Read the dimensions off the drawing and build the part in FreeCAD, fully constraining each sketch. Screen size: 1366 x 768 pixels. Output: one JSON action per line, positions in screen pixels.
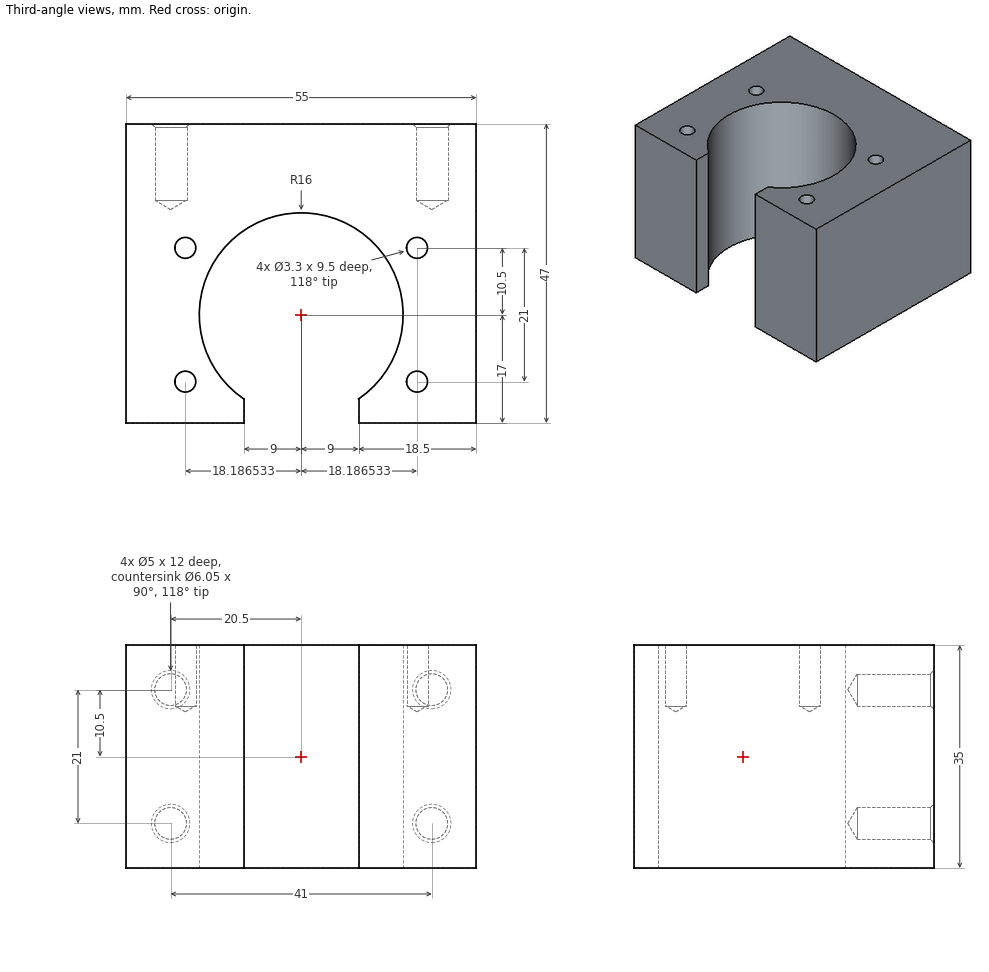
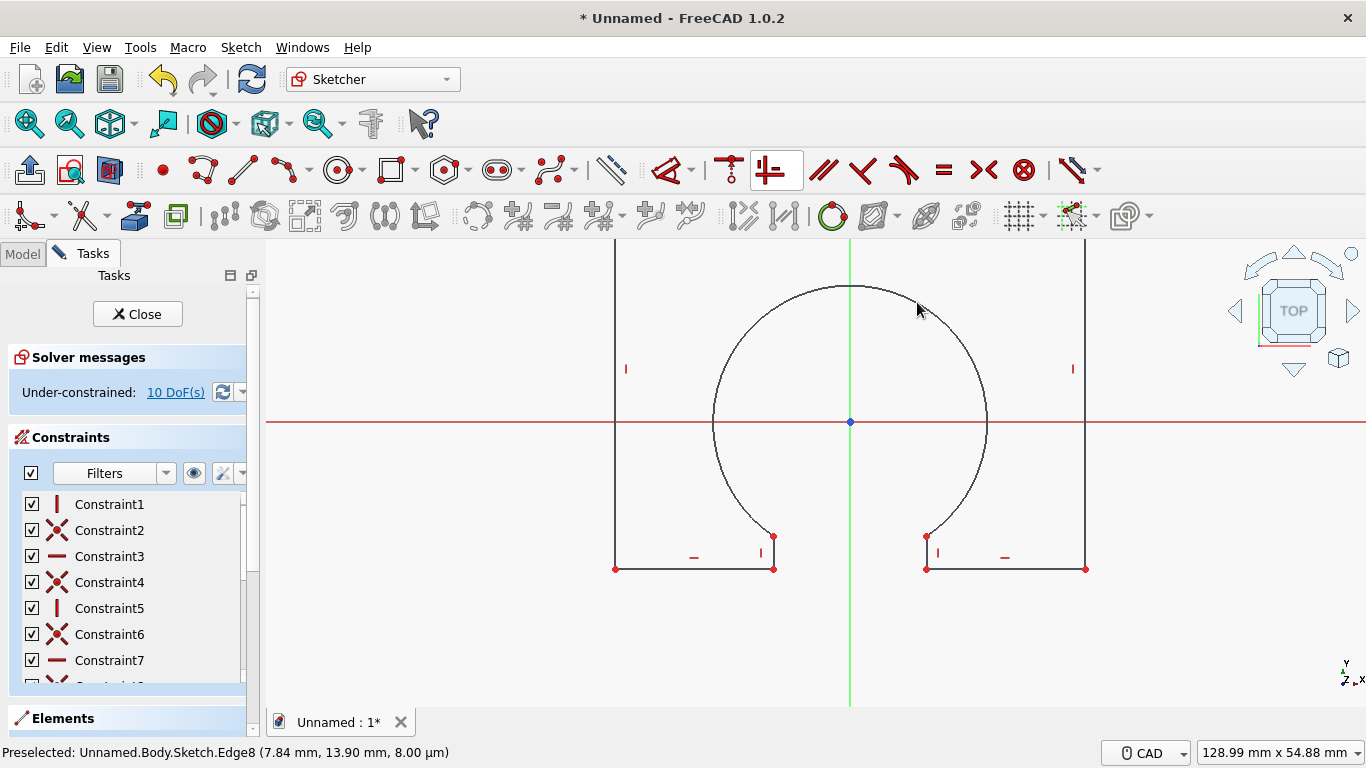
{"action": "left_click_drag", "start_coordinate": [840, 412], "coordinate": [860, 433]}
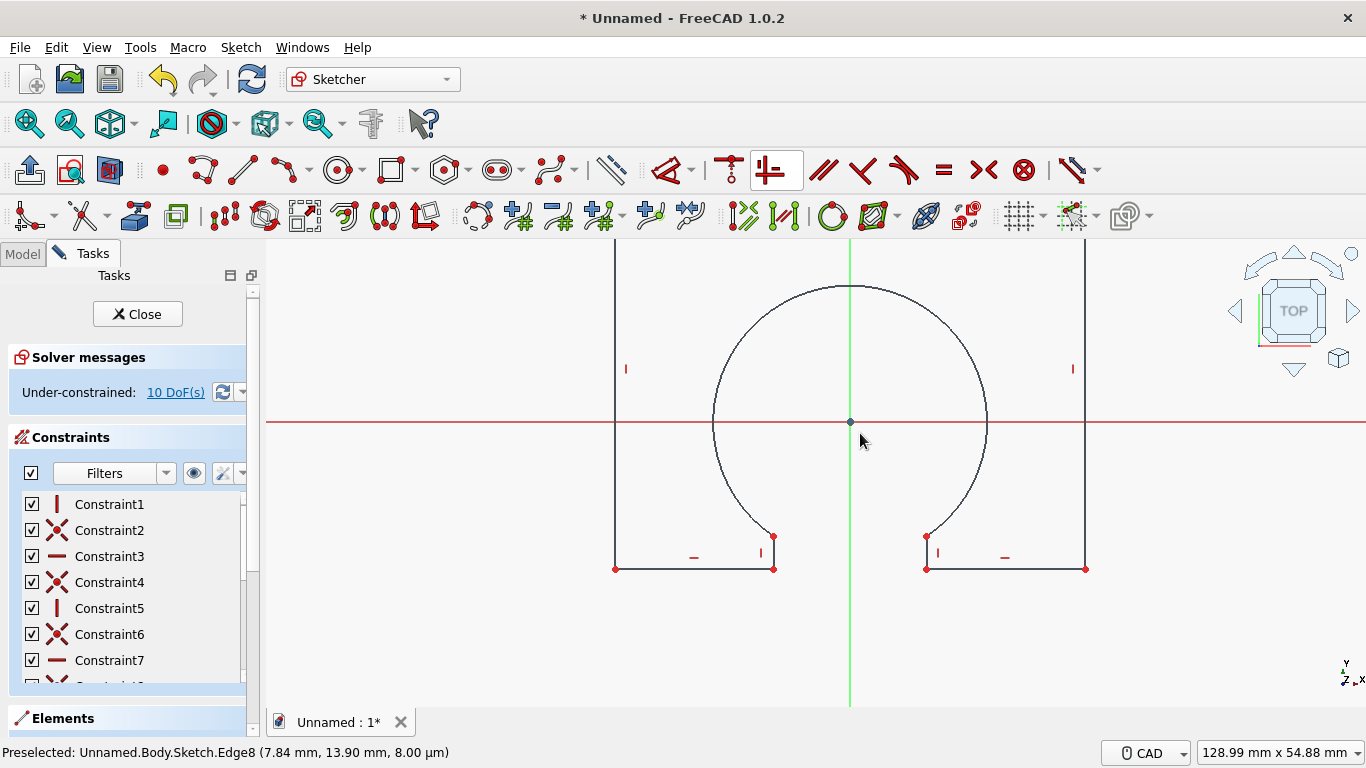
{"action": "left_click", "coordinate": [730, 170]}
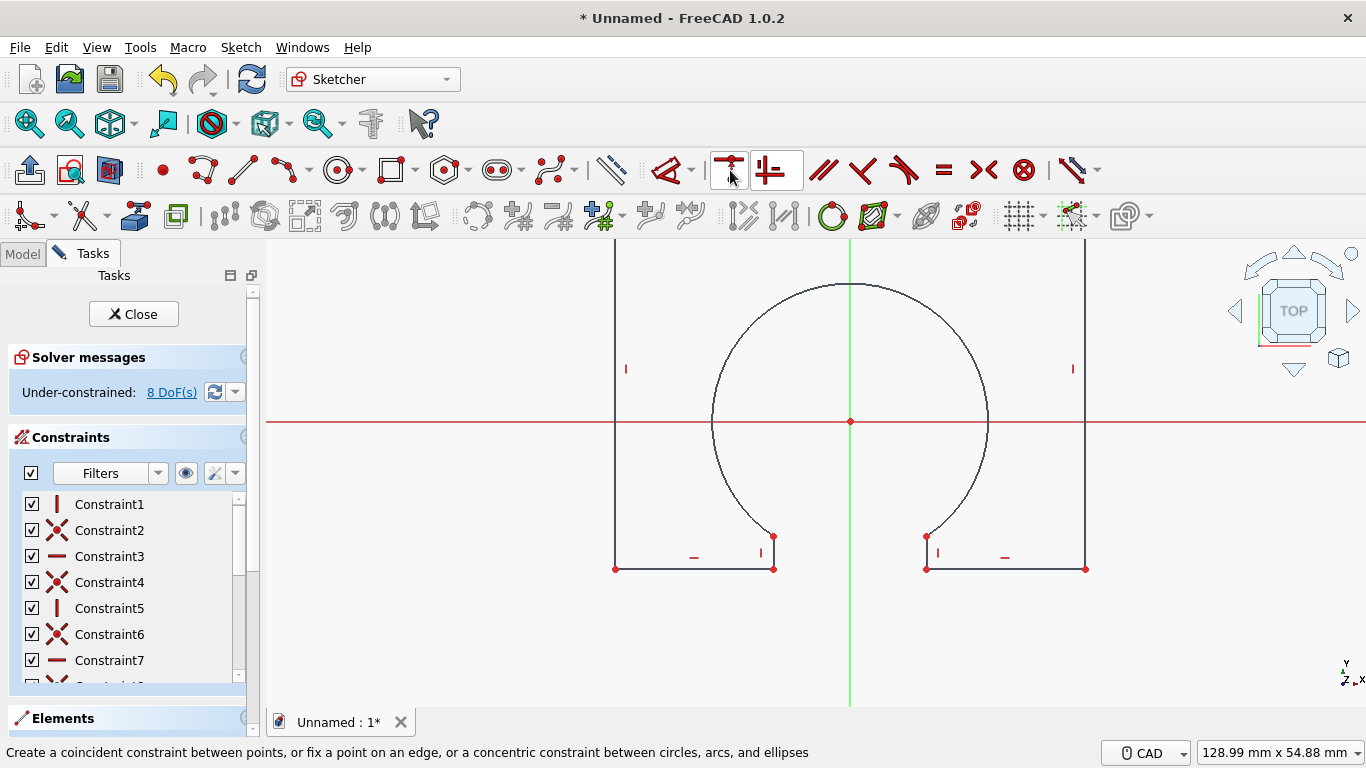
{"action": "left_click", "coordinate": [666, 170]}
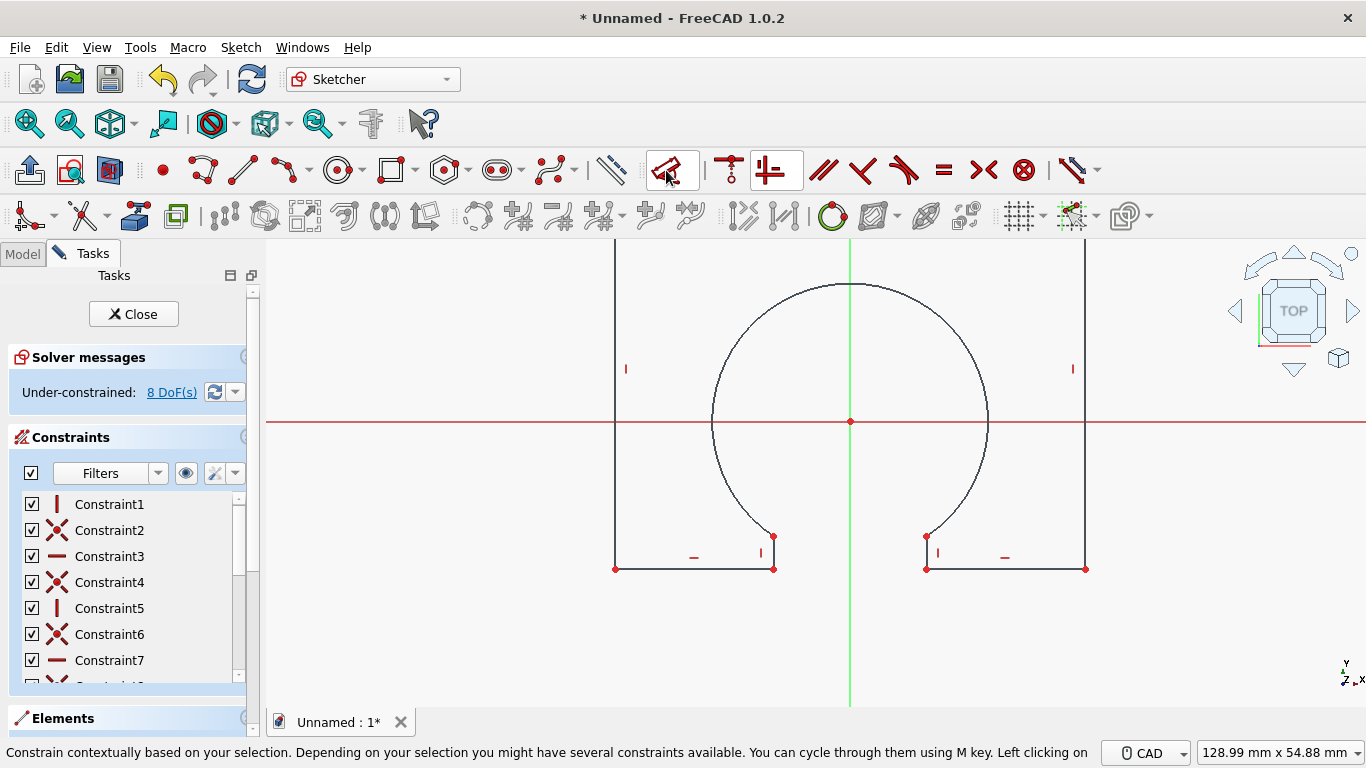
{"action": "left_click", "coordinate": [968, 349]}
{"action": "left_click", "coordinate": [995, 332]}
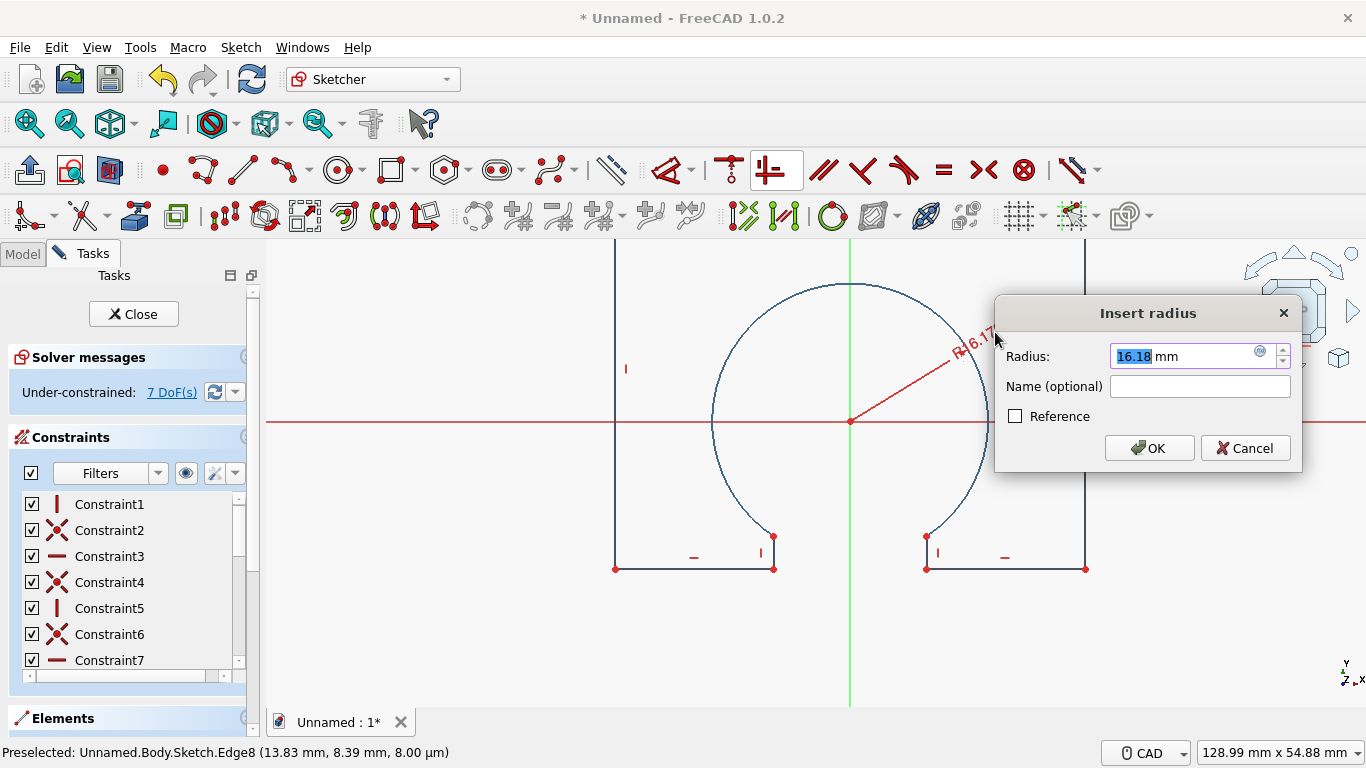
{"action": "type", "text": "16"}
{"action": "key", "text": "Return"}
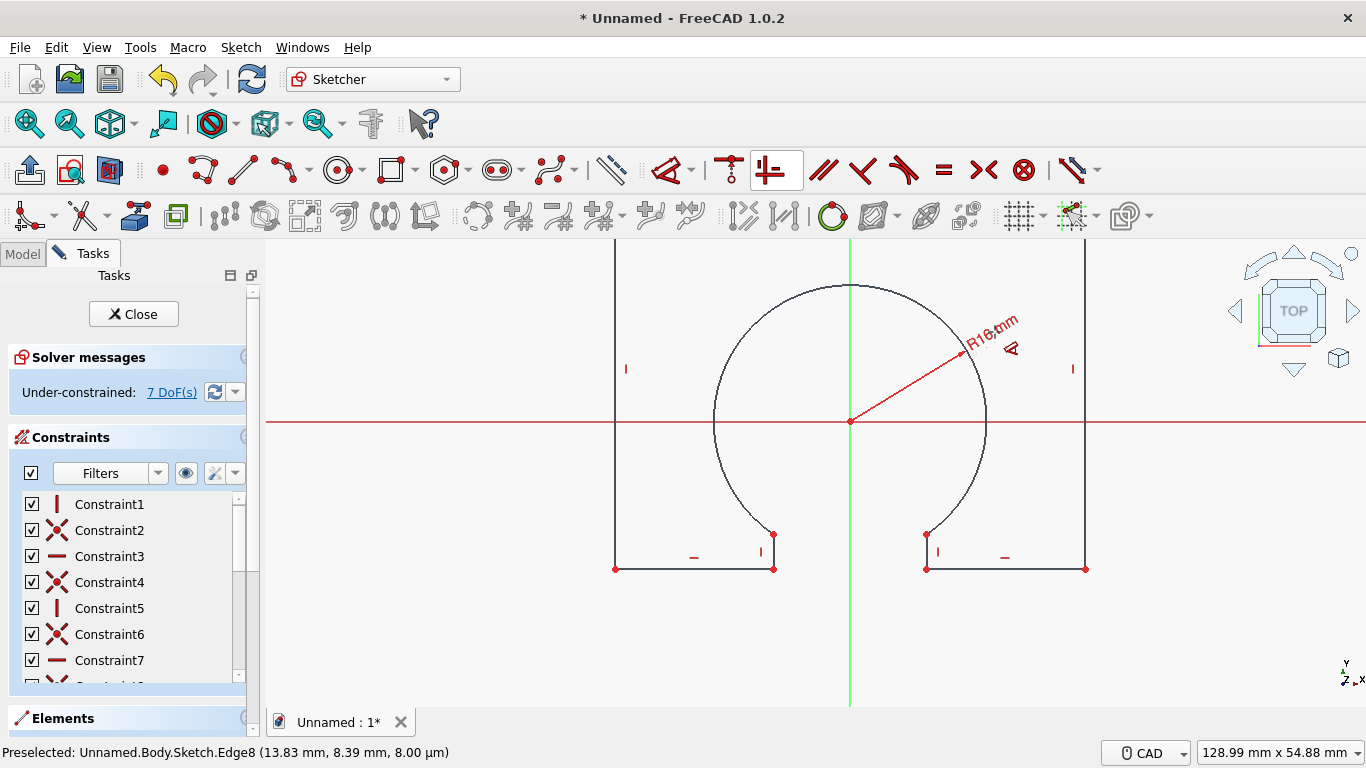
{"action": "left_click", "coordinate": [1085, 449]}
{"action": "left_click", "coordinate": [1119, 349]}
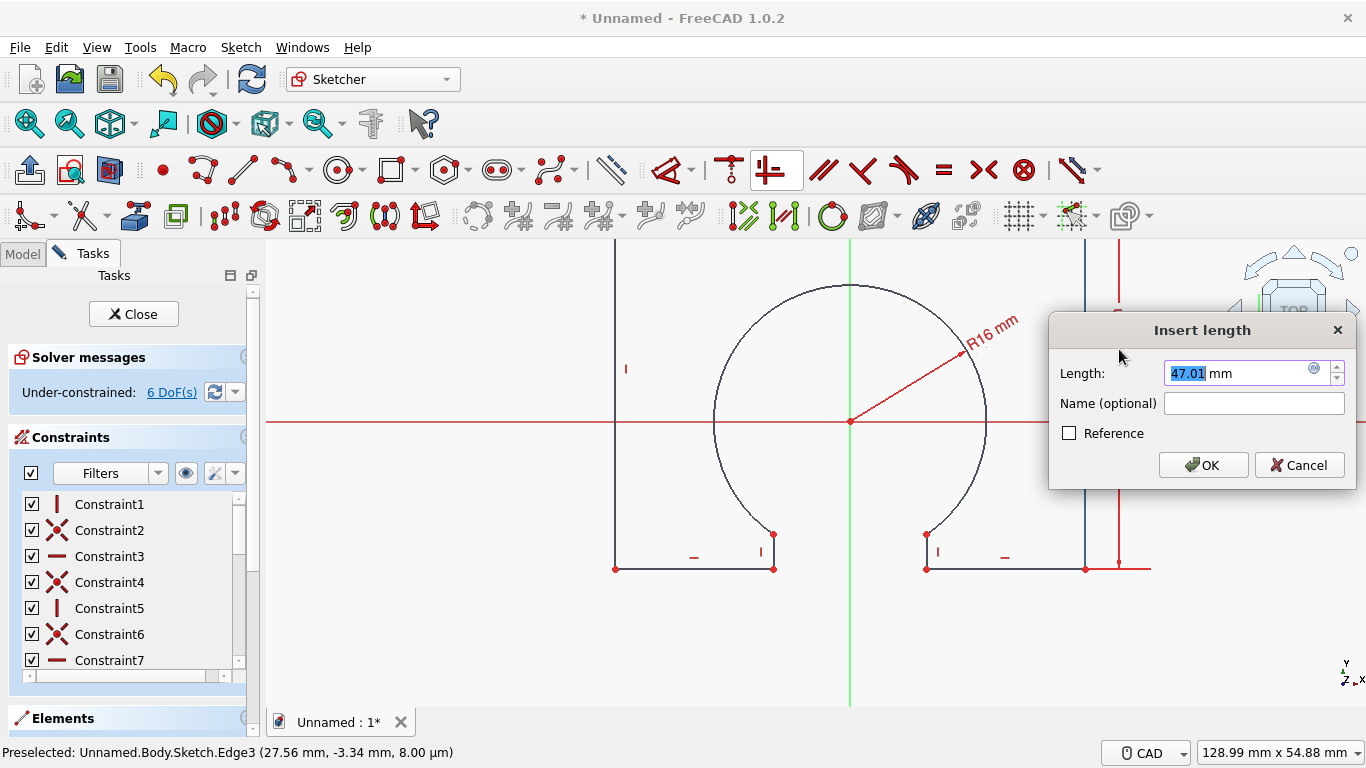
{"action": "type", "text": "47"}
{"action": "key", "text": "Return"}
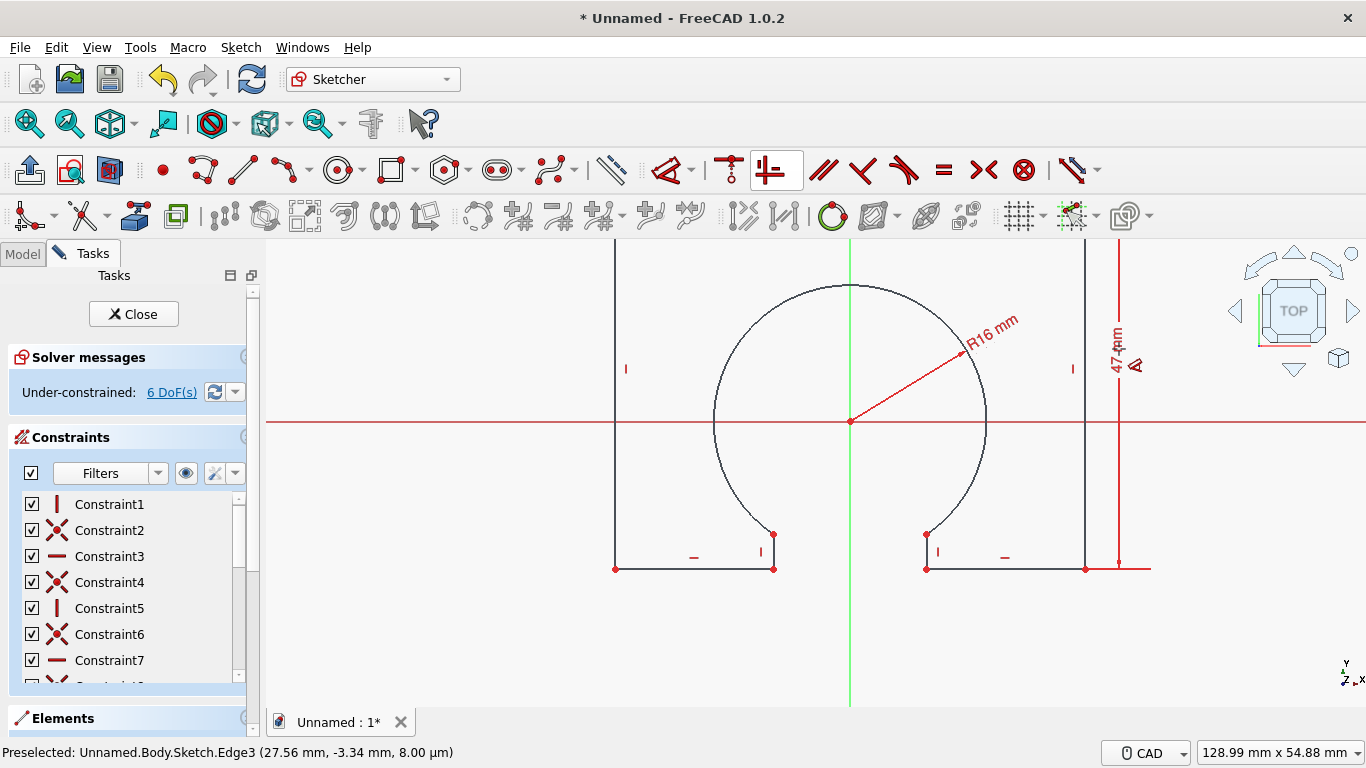
{"action": "scroll", "coordinate": [539, 679], "scroll_direction": "down", "scroll_amount": 2}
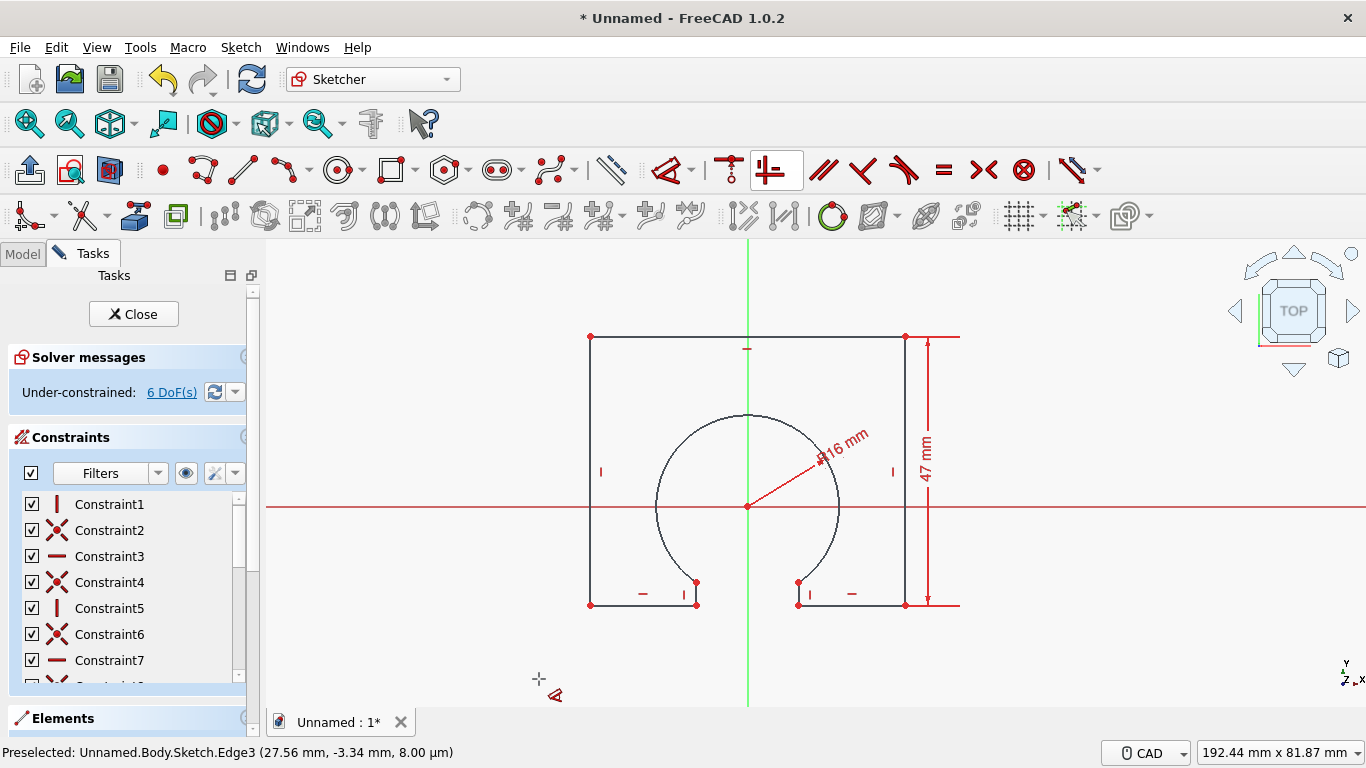
{"action": "left_click", "coordinate": [811, 337]}
{"action": "left_click", "coordinate": [675, 303]}